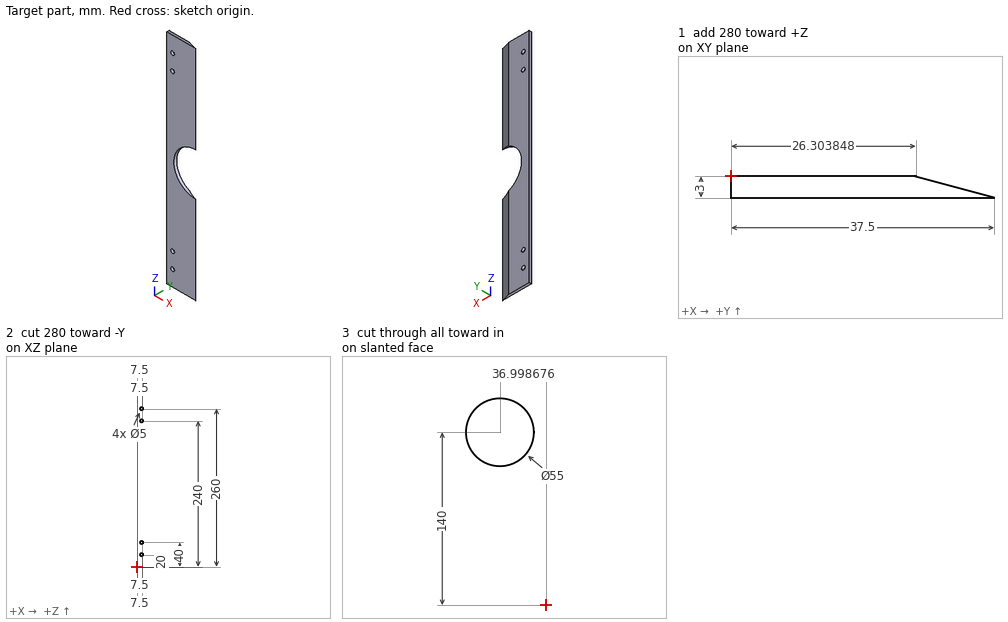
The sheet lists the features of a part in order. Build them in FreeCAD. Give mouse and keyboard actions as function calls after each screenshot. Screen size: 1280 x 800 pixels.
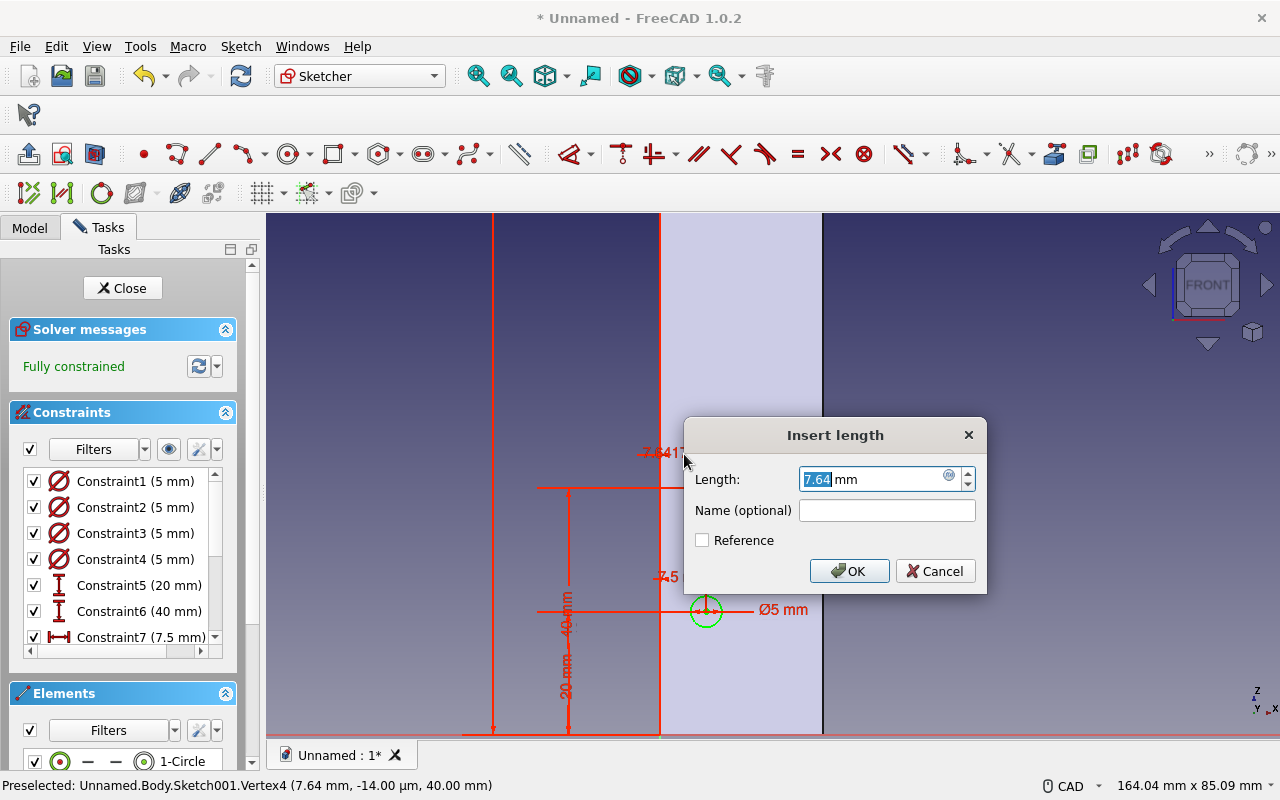
text(7.5)
key(Return)
key(Escape)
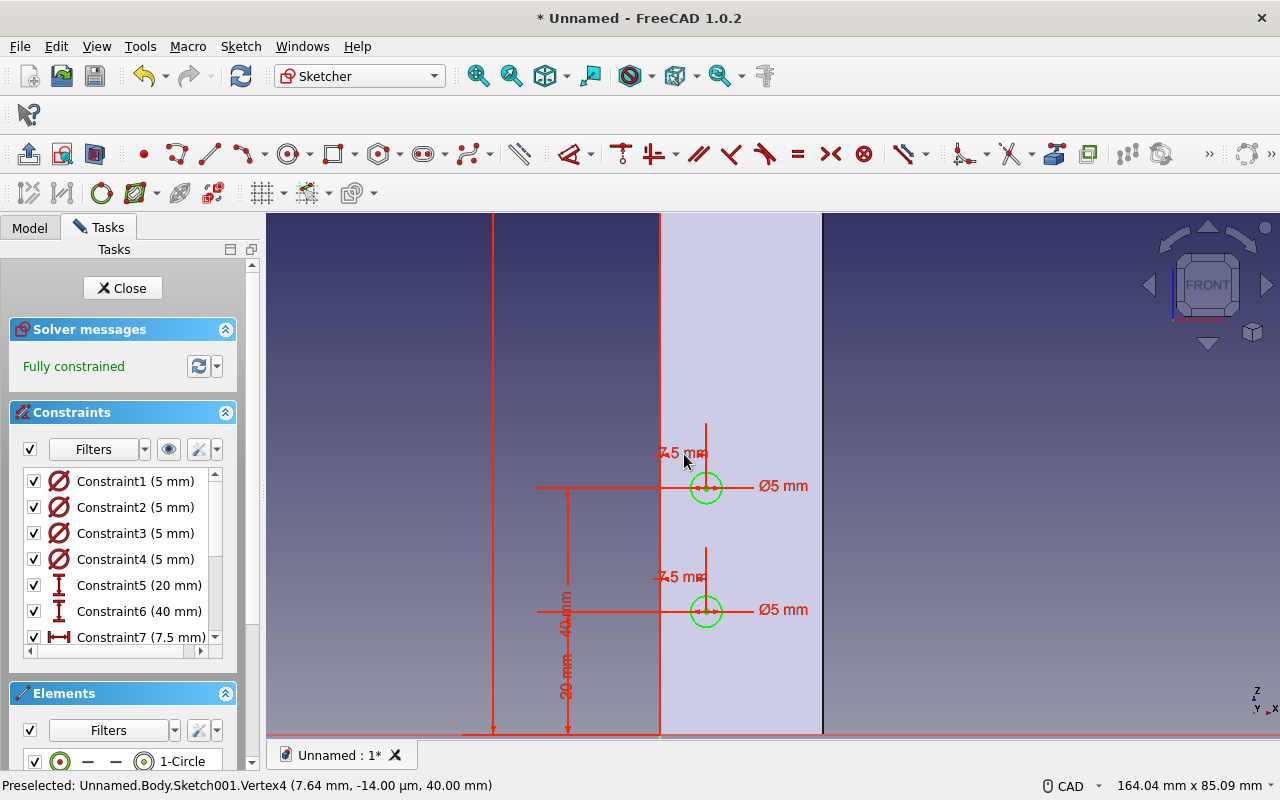
click(123, 288)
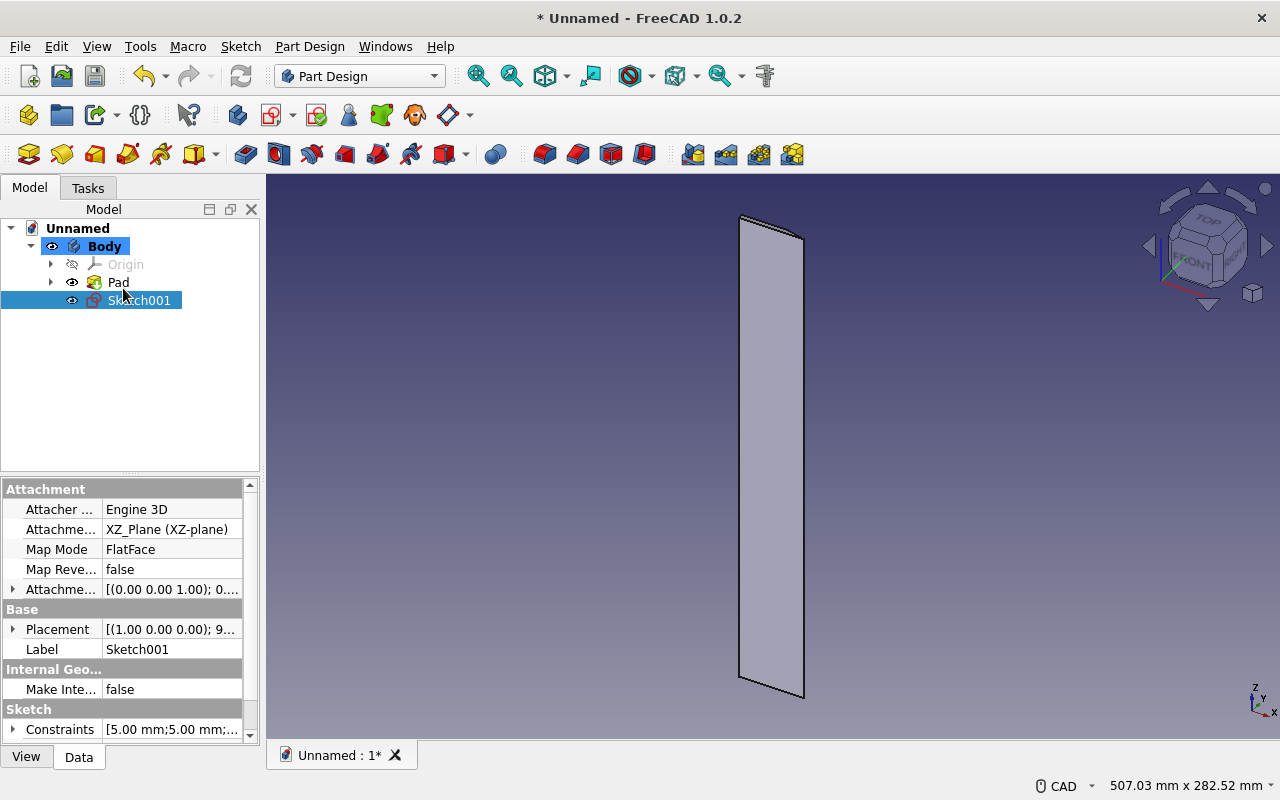
click(246, 154)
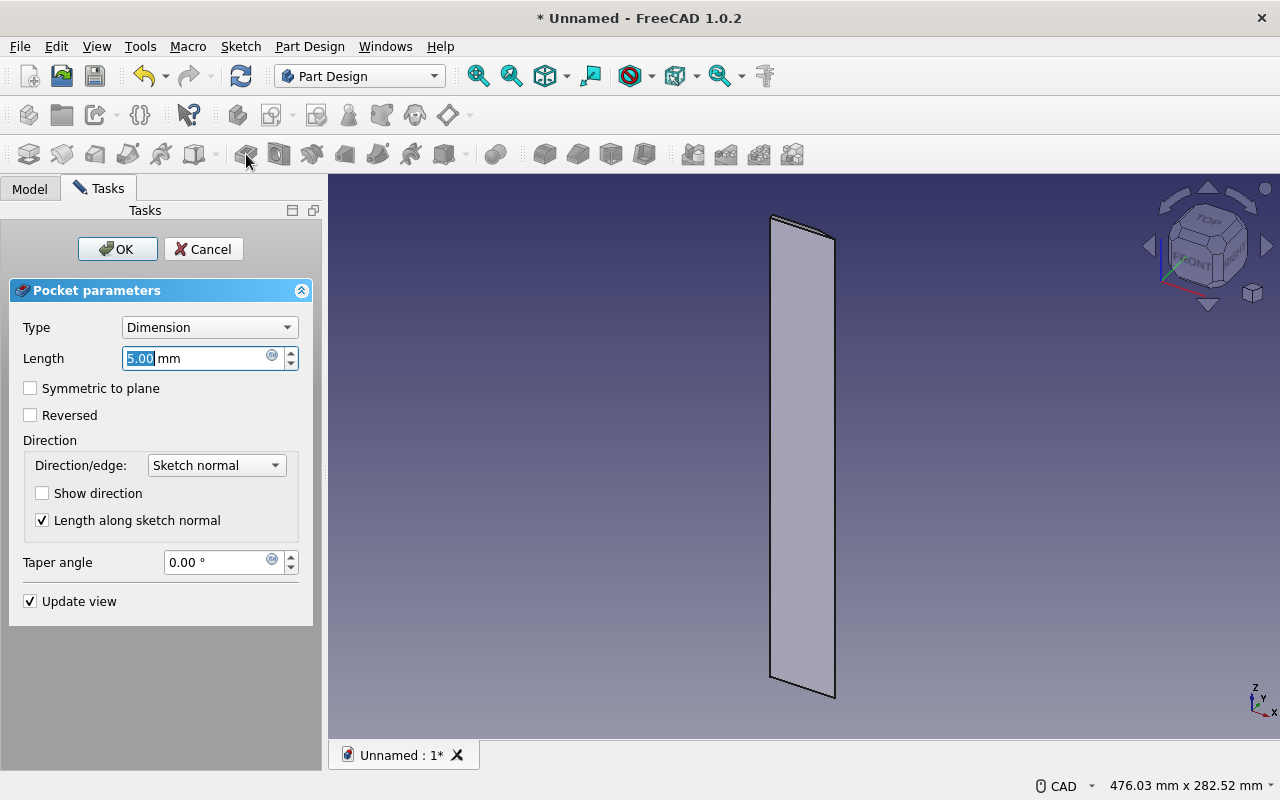
text(280)
key(Tab)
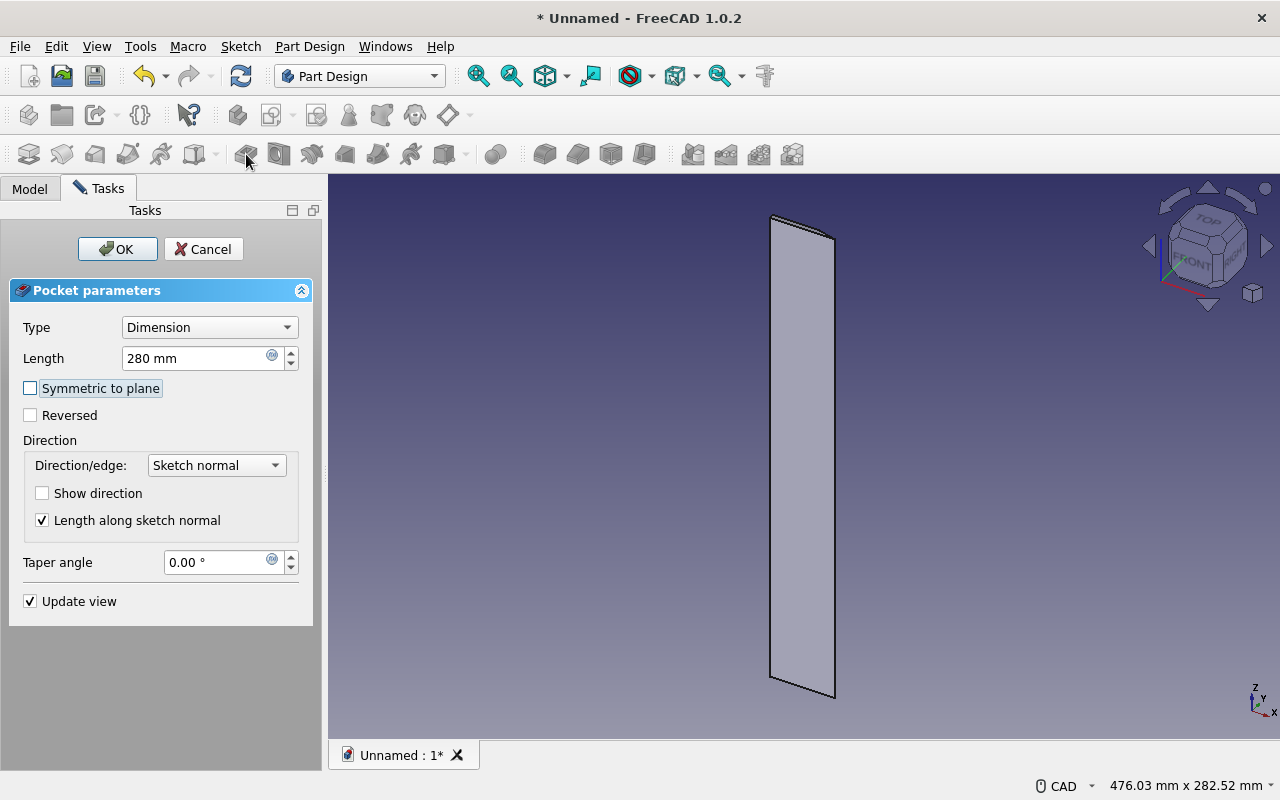
click(31, 415)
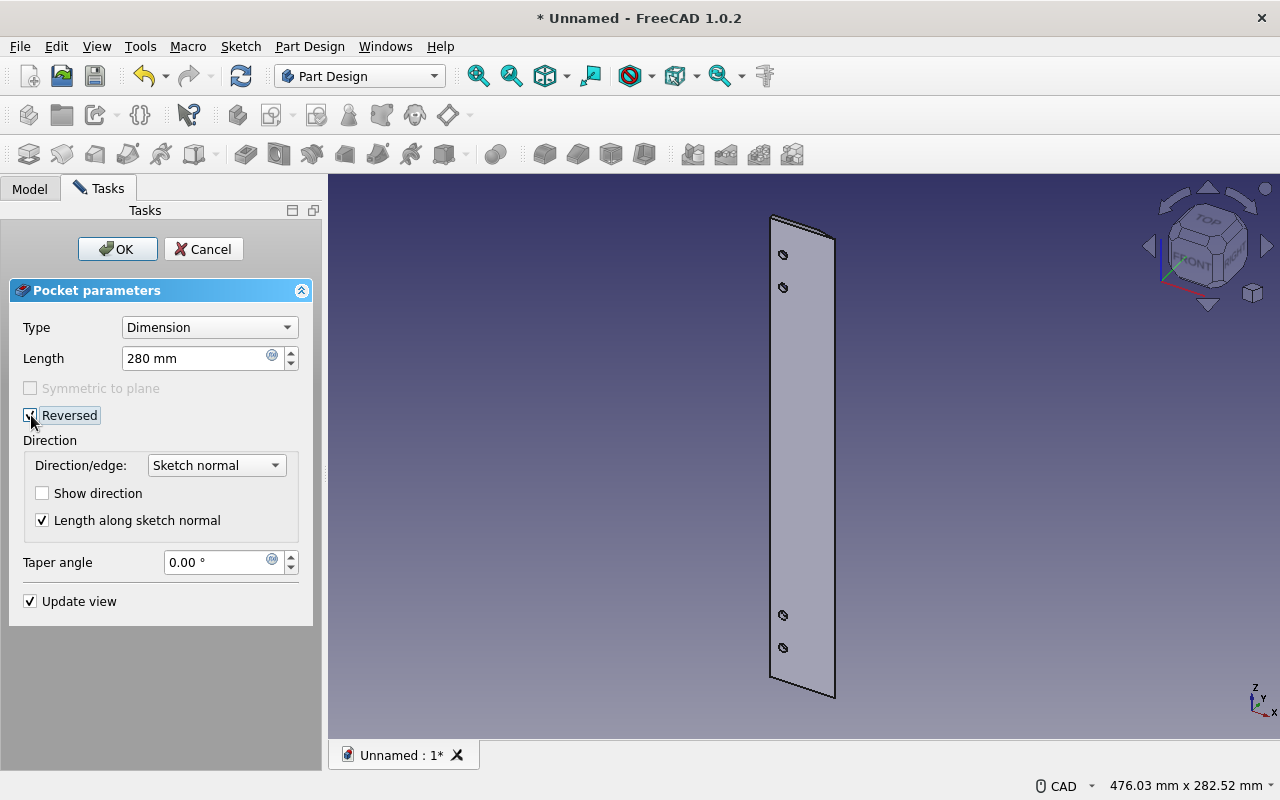
click(118, 249)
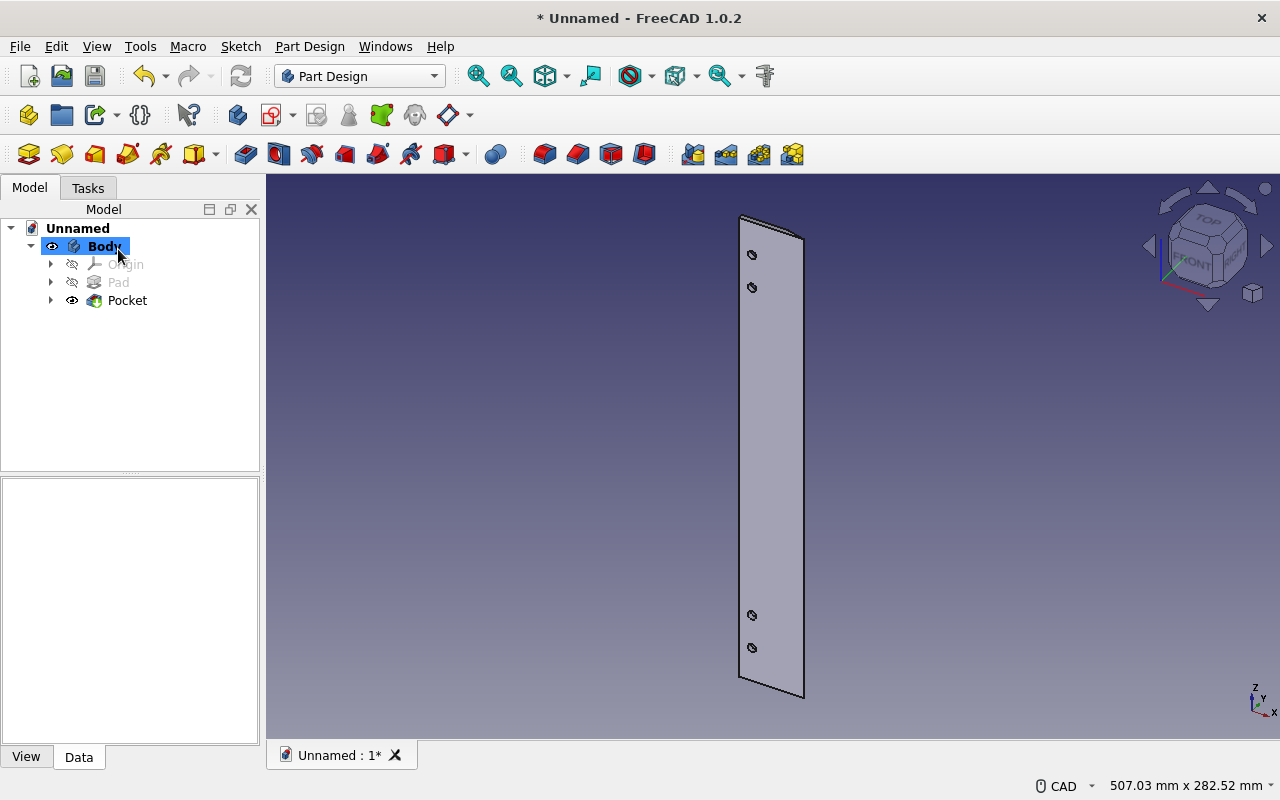
key(4)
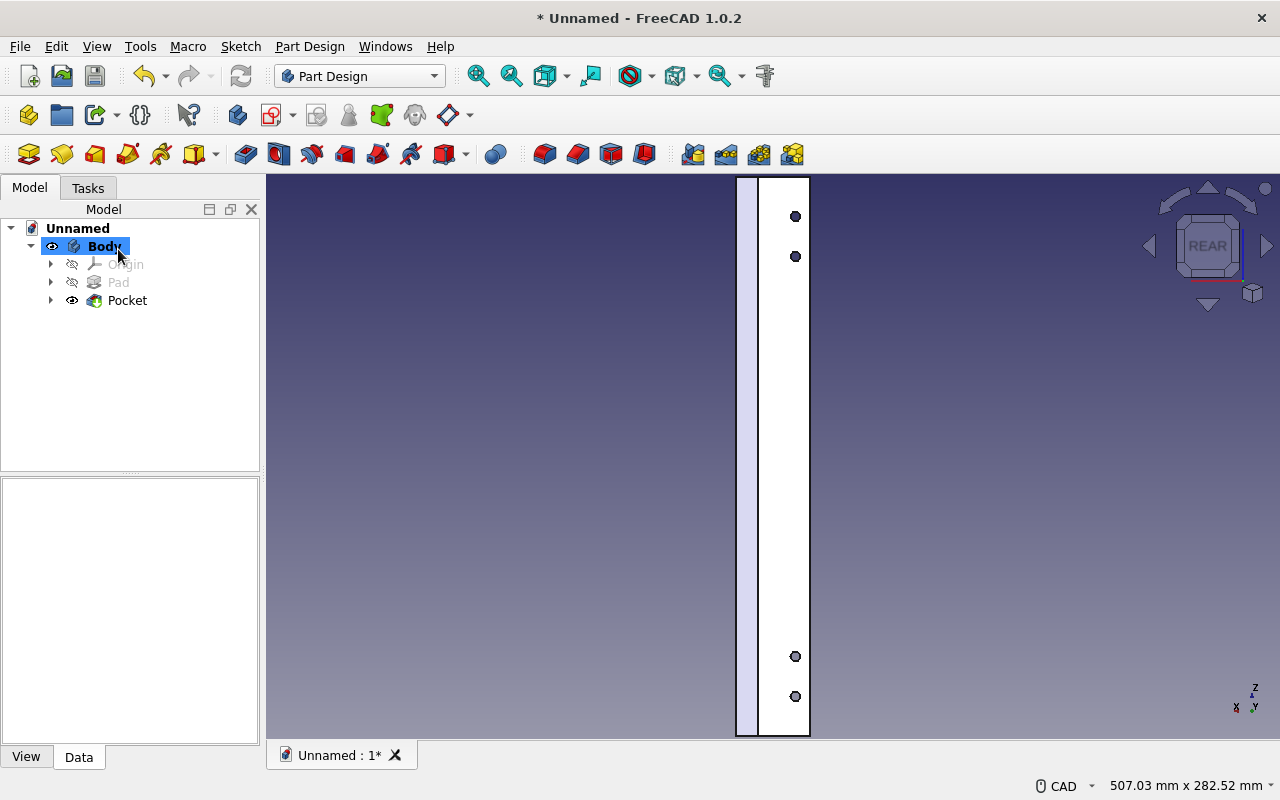
click(747, 216)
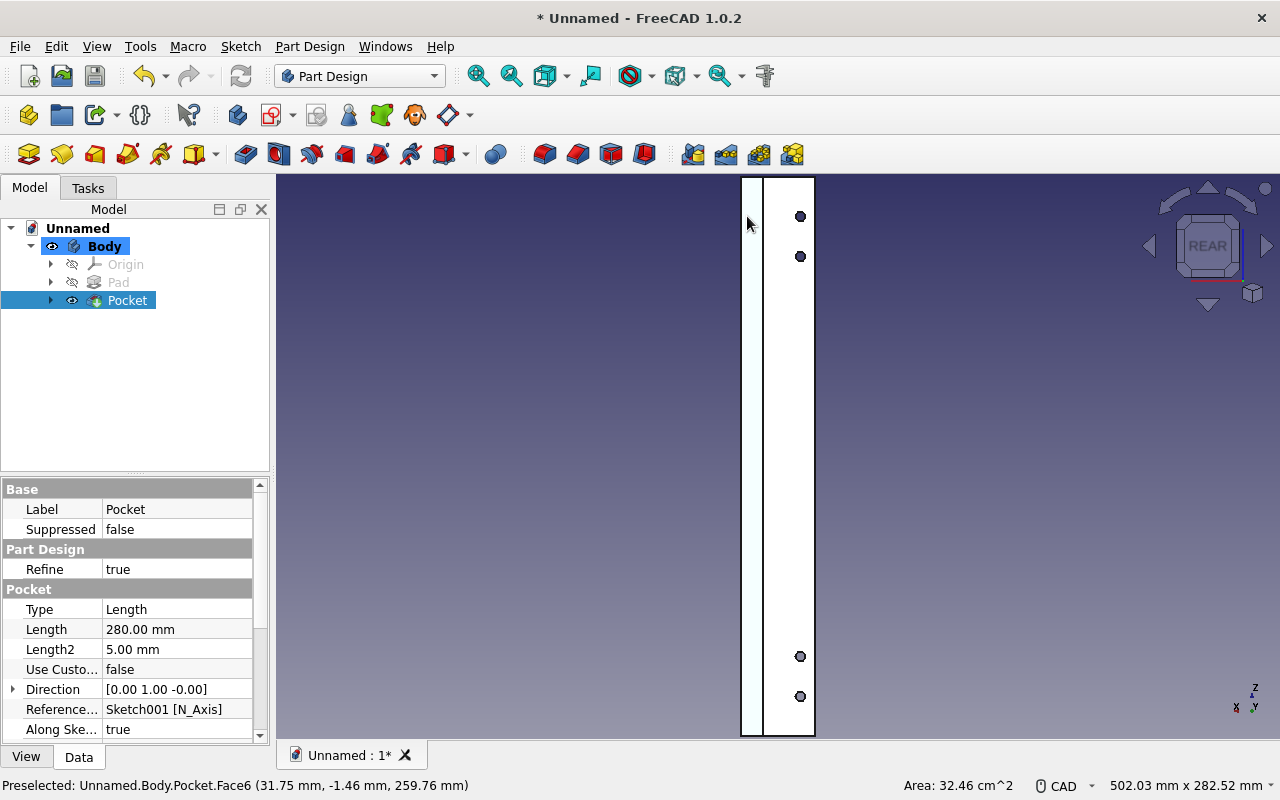
click(270, 116)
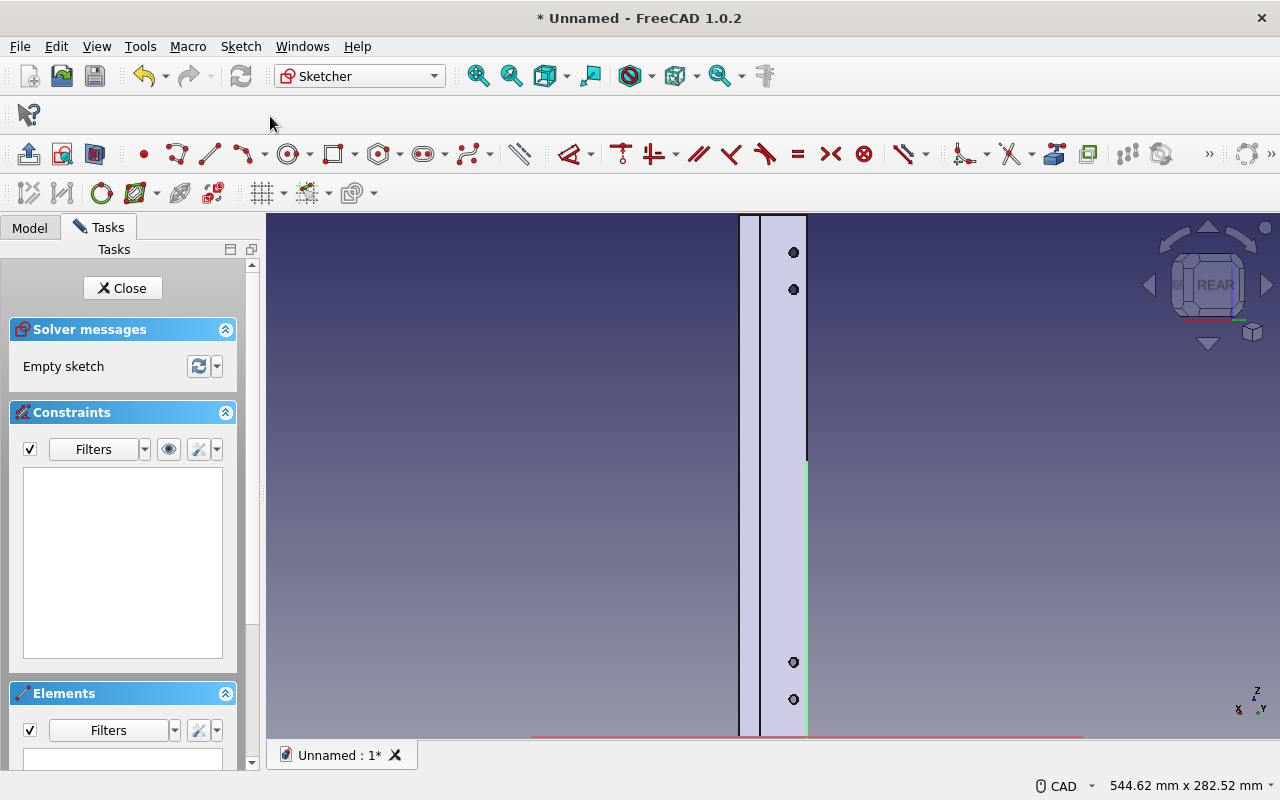
click(95, 154)